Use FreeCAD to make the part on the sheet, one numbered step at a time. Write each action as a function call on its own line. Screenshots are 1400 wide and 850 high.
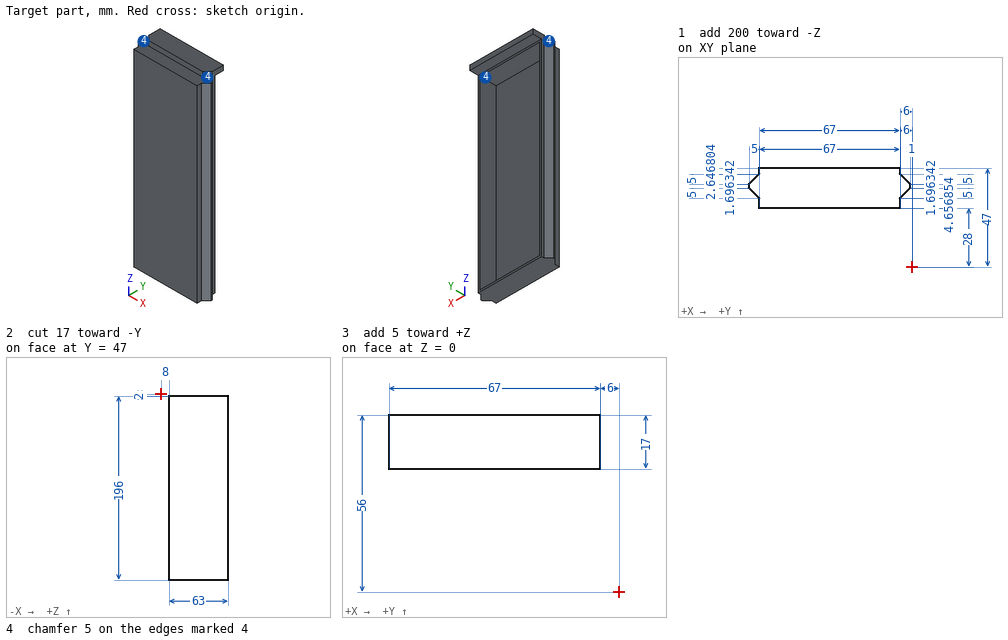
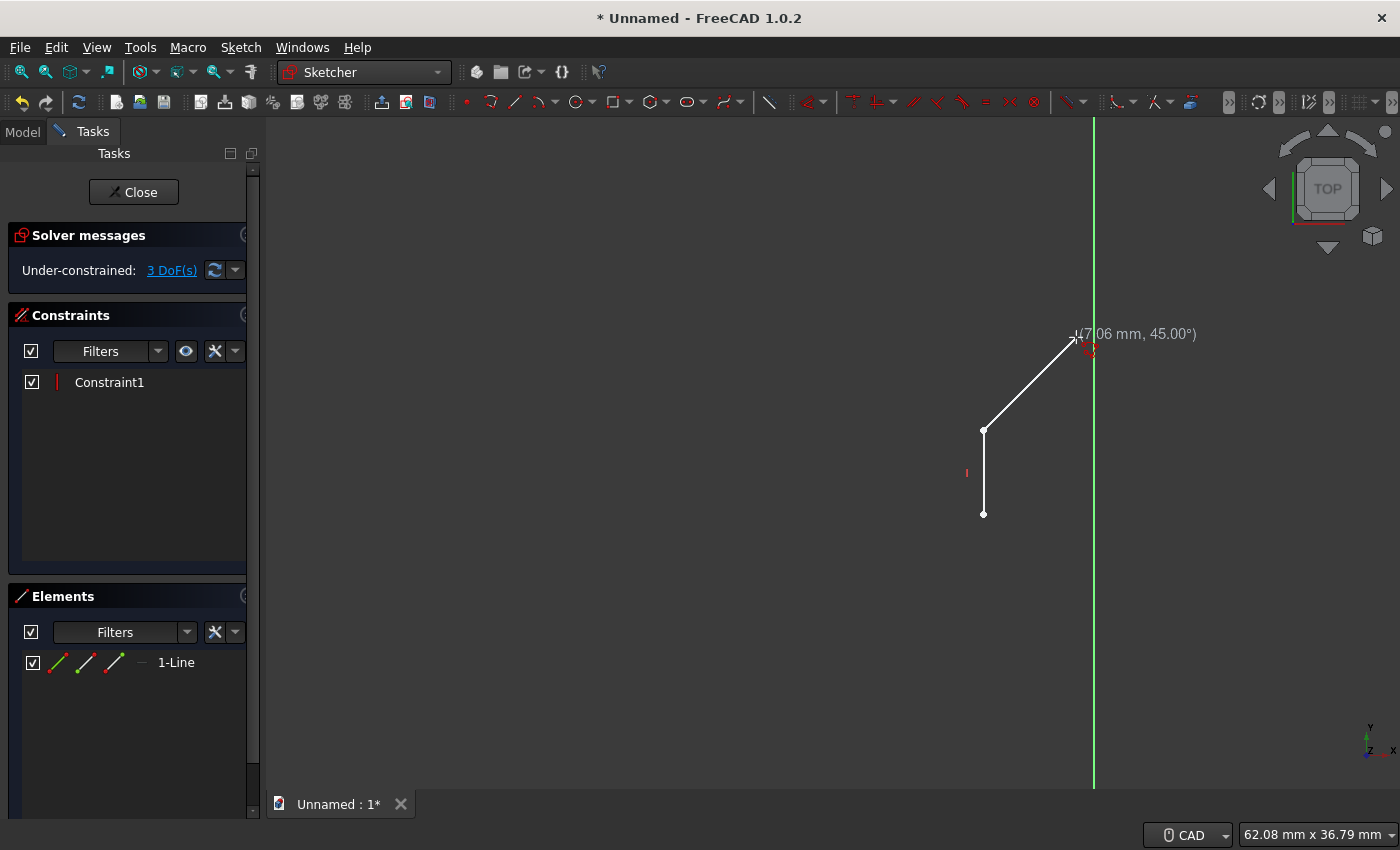
click(1076, 336)
click(1076, 305)
click(984, 213)
click(984, 165)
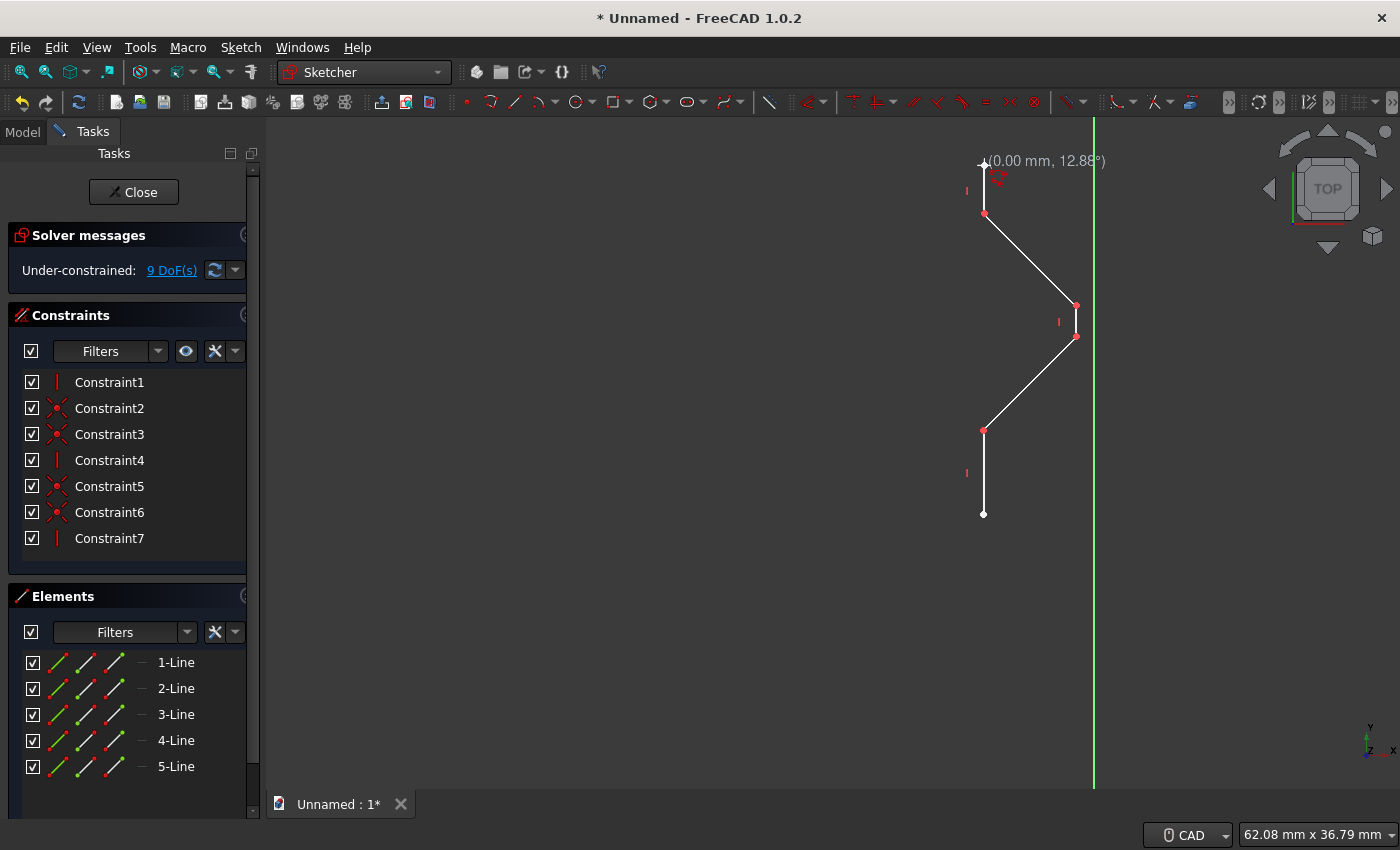
scroll(1077, 338, down, 4)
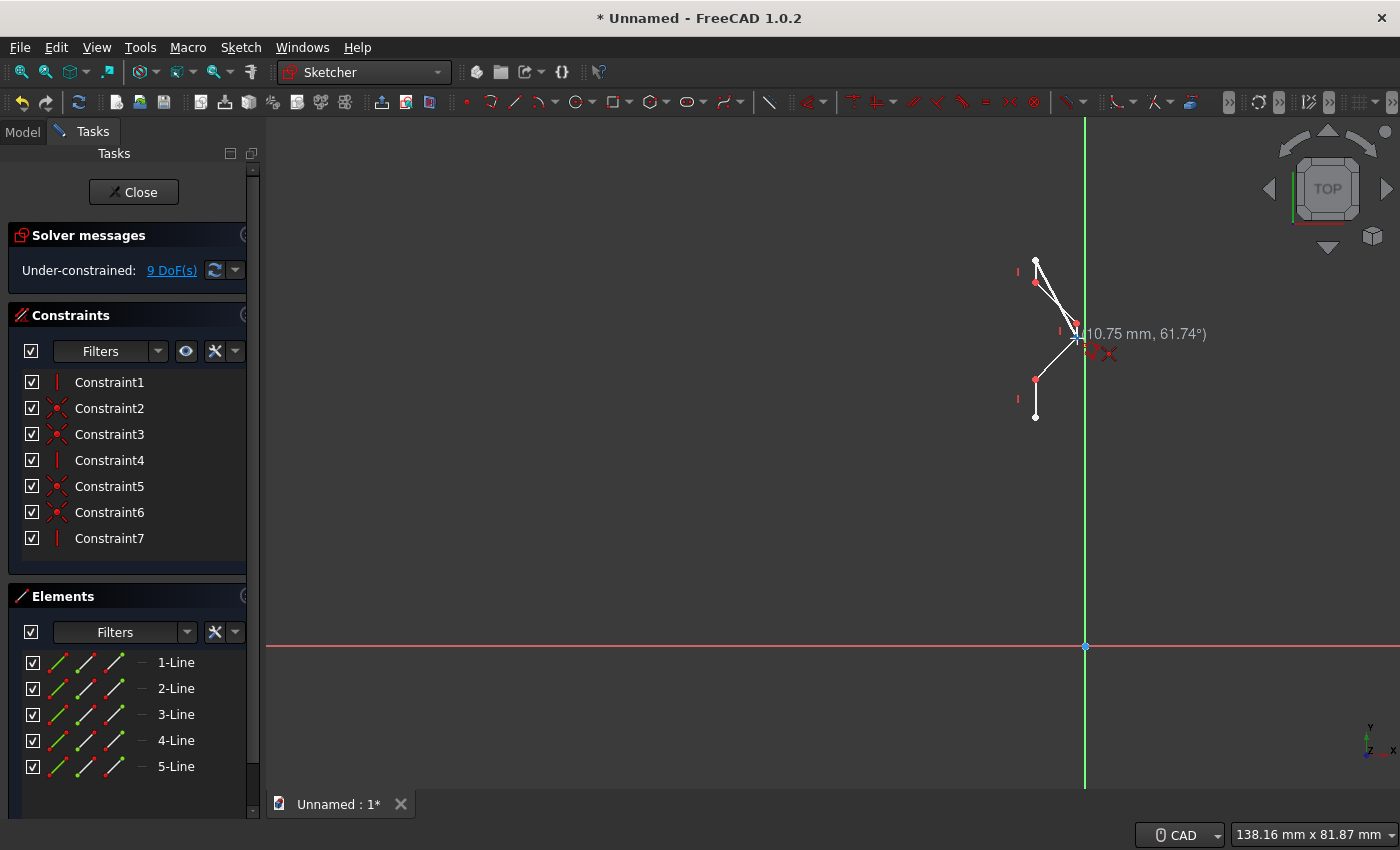
click(486, 260)
click(486, 282)
click(445, 323)
click(445, 337)
click(486, 378)
click(486, 416)
click(1036, 418)
key(Escape)
key(Escape)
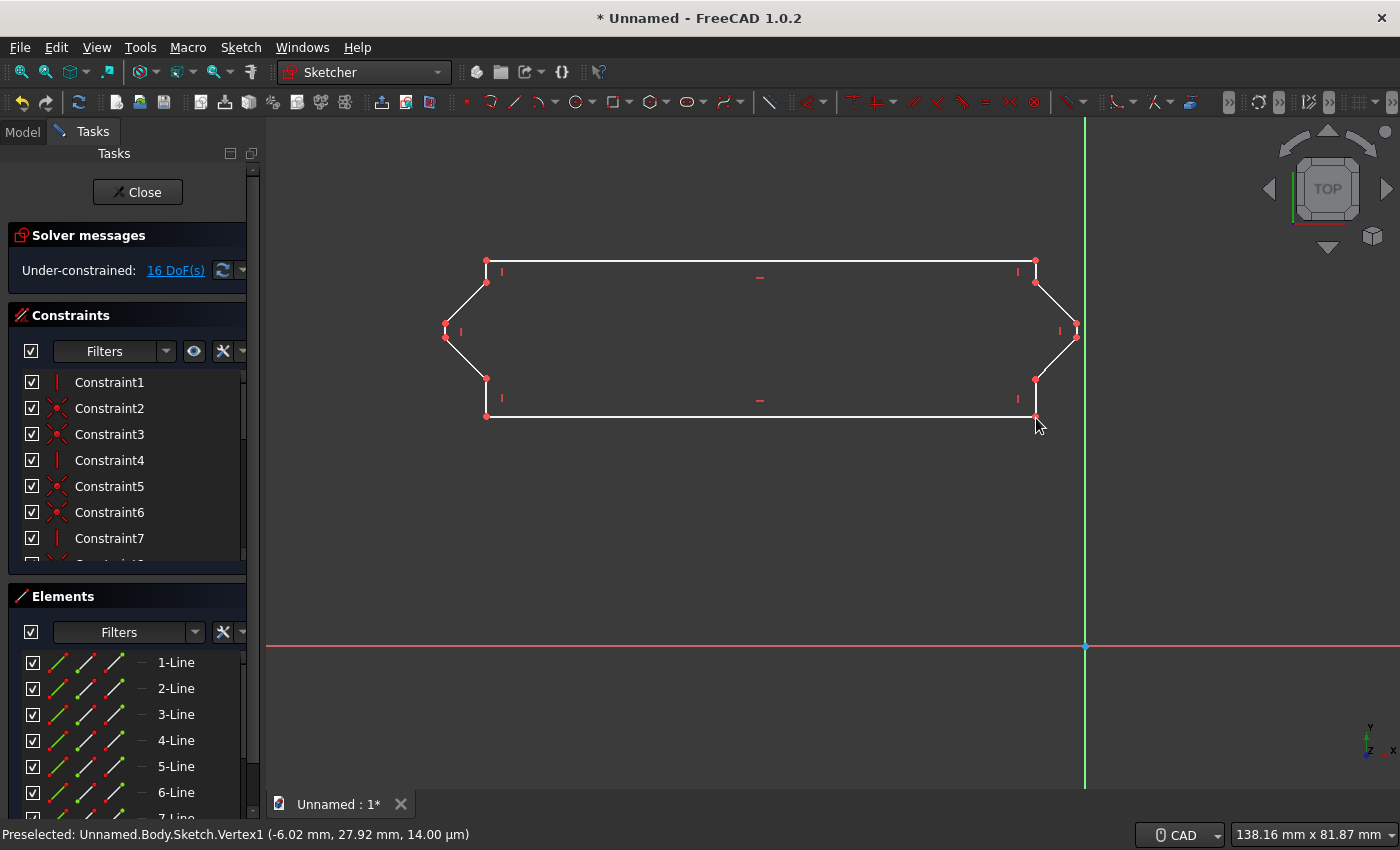
key(d)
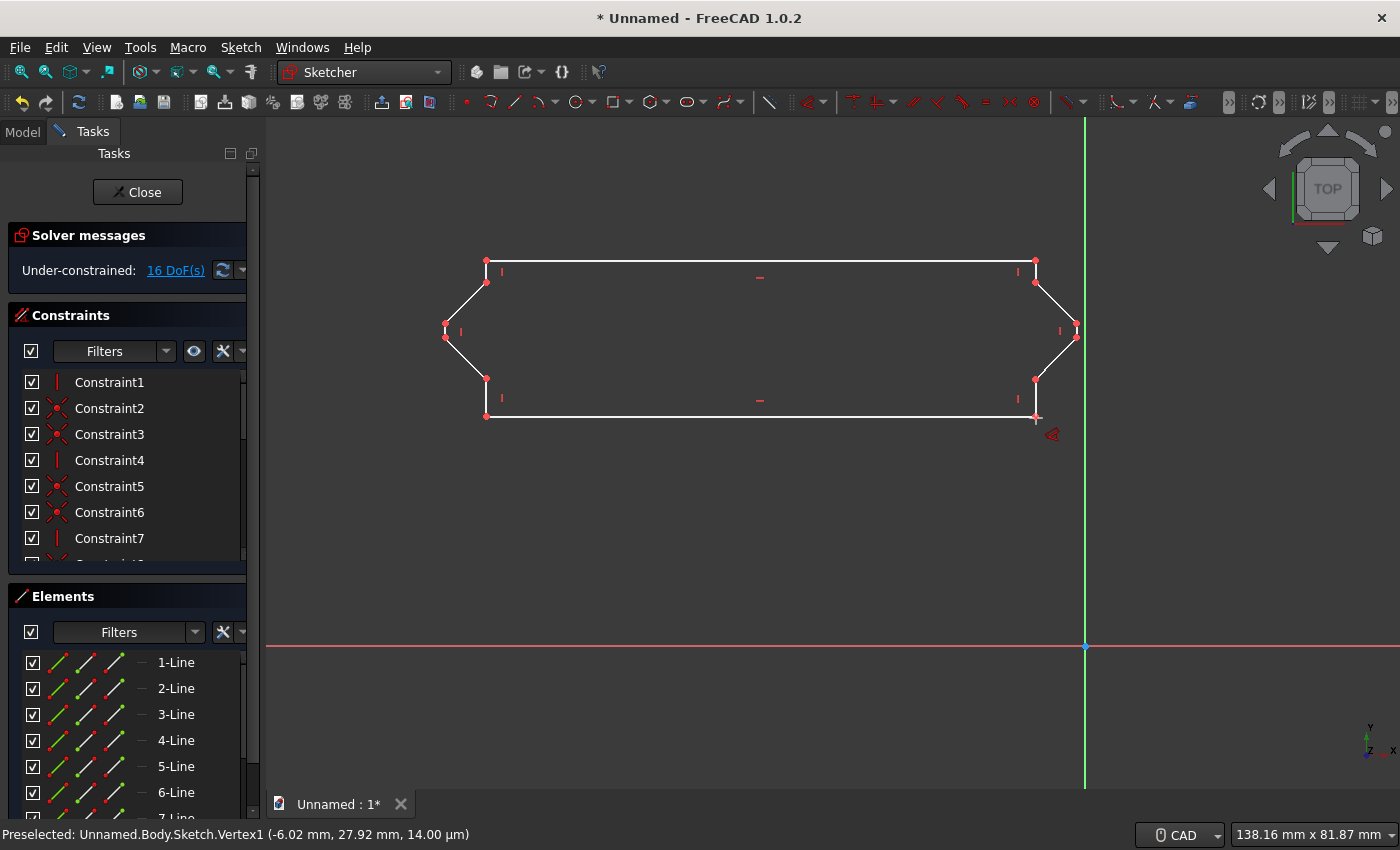
click(871, 261)
click(761, 227)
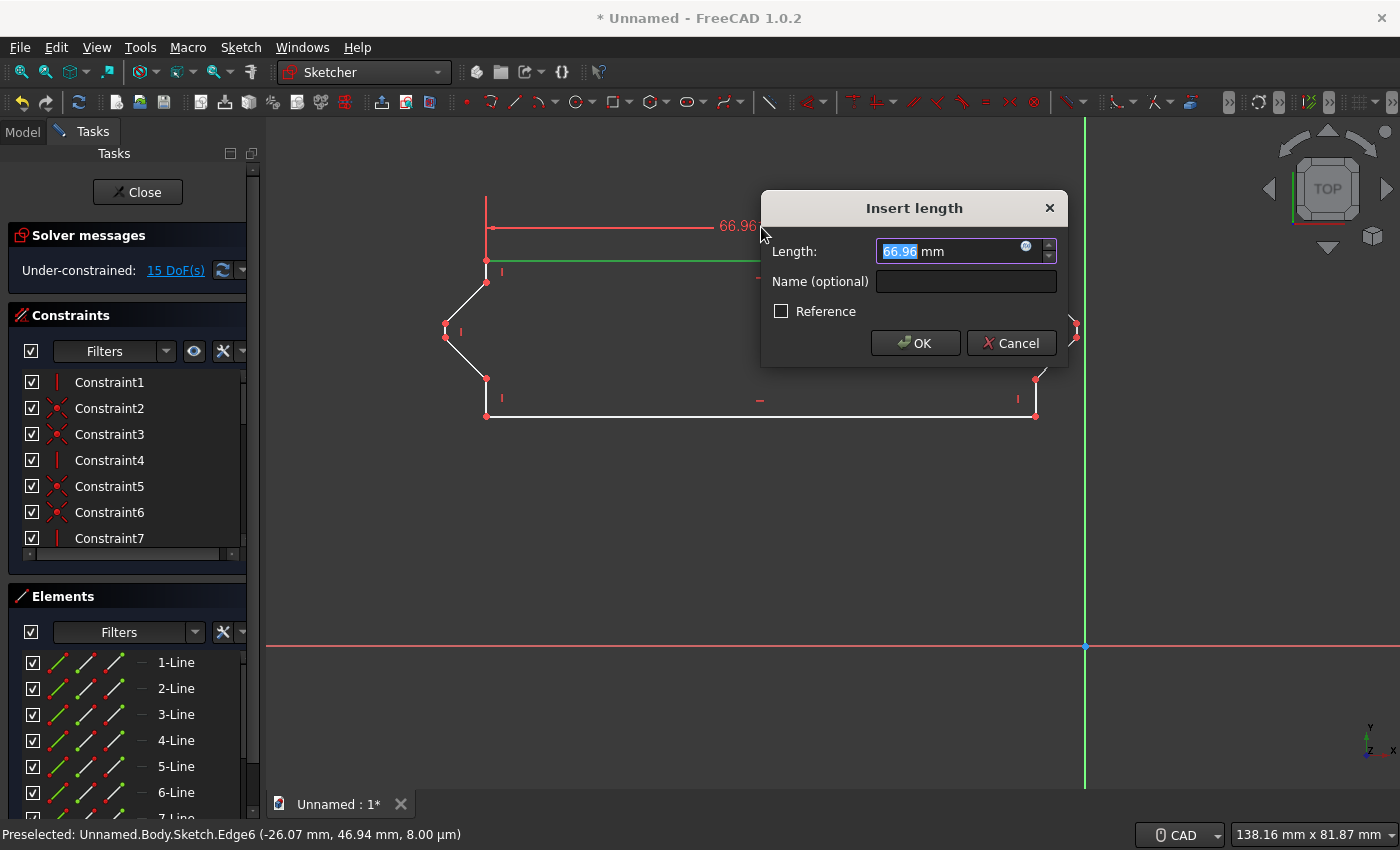
text(67)
key(Return)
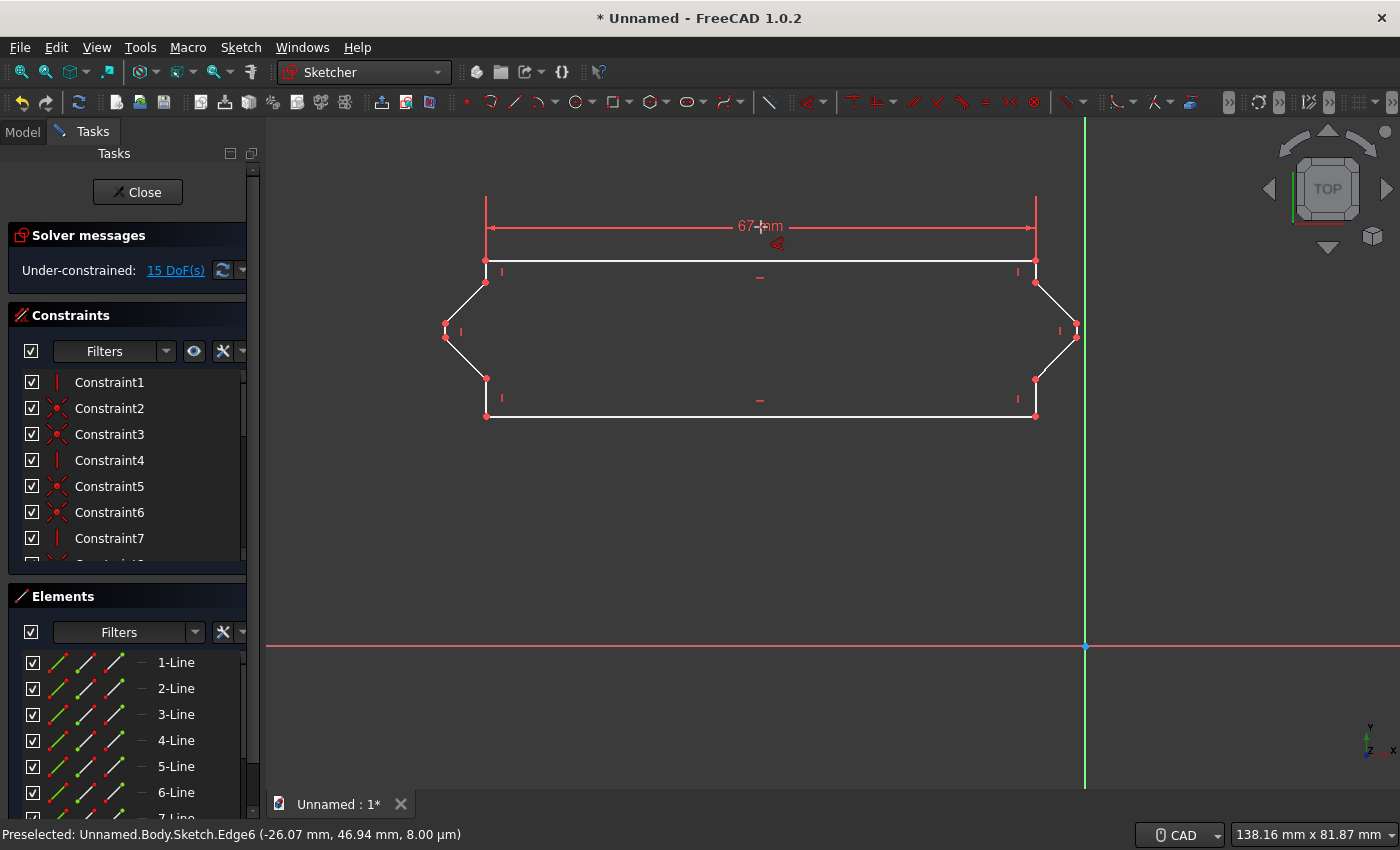
click(651, 417)
click(761, 383)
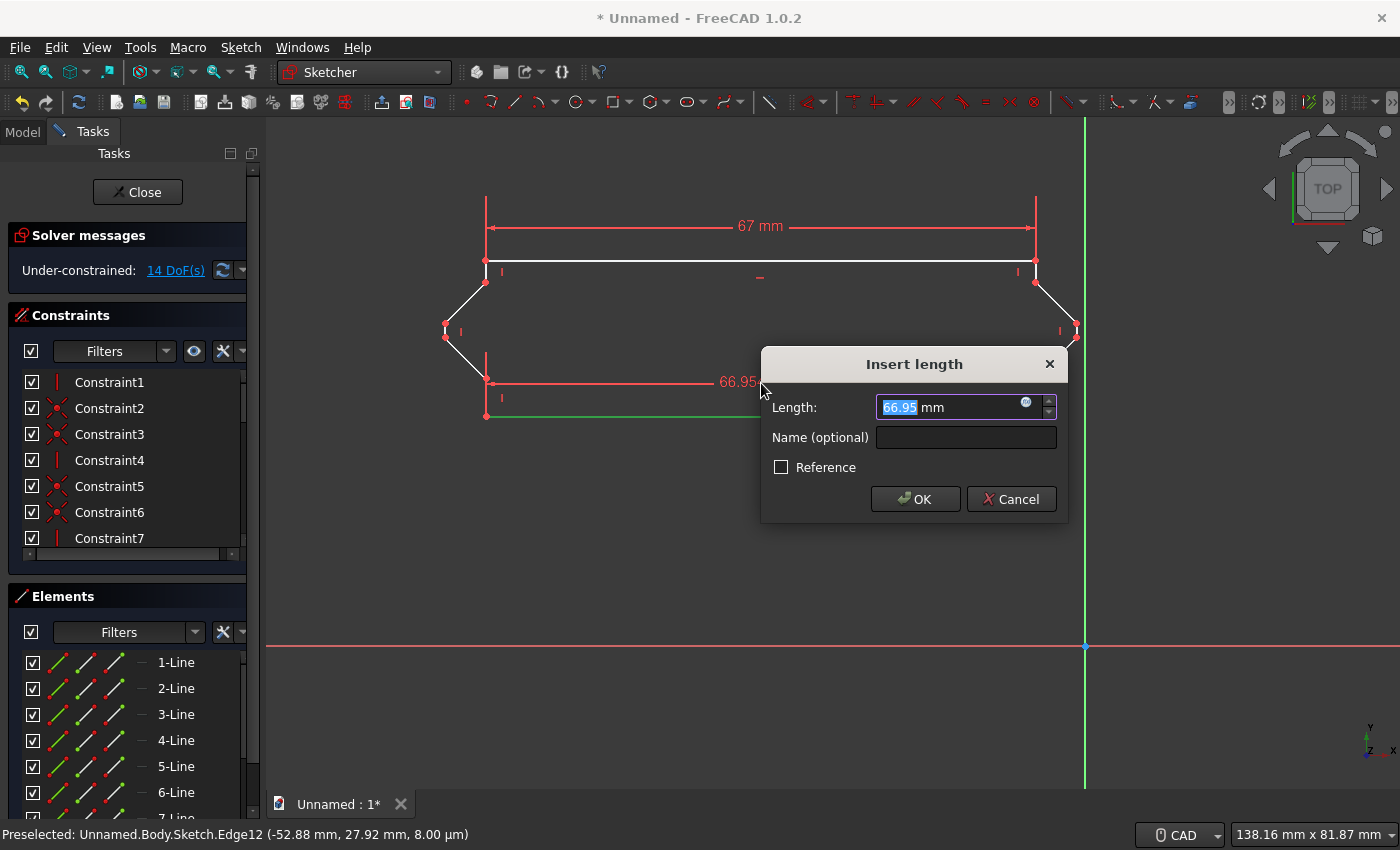
text(67)
key(Return)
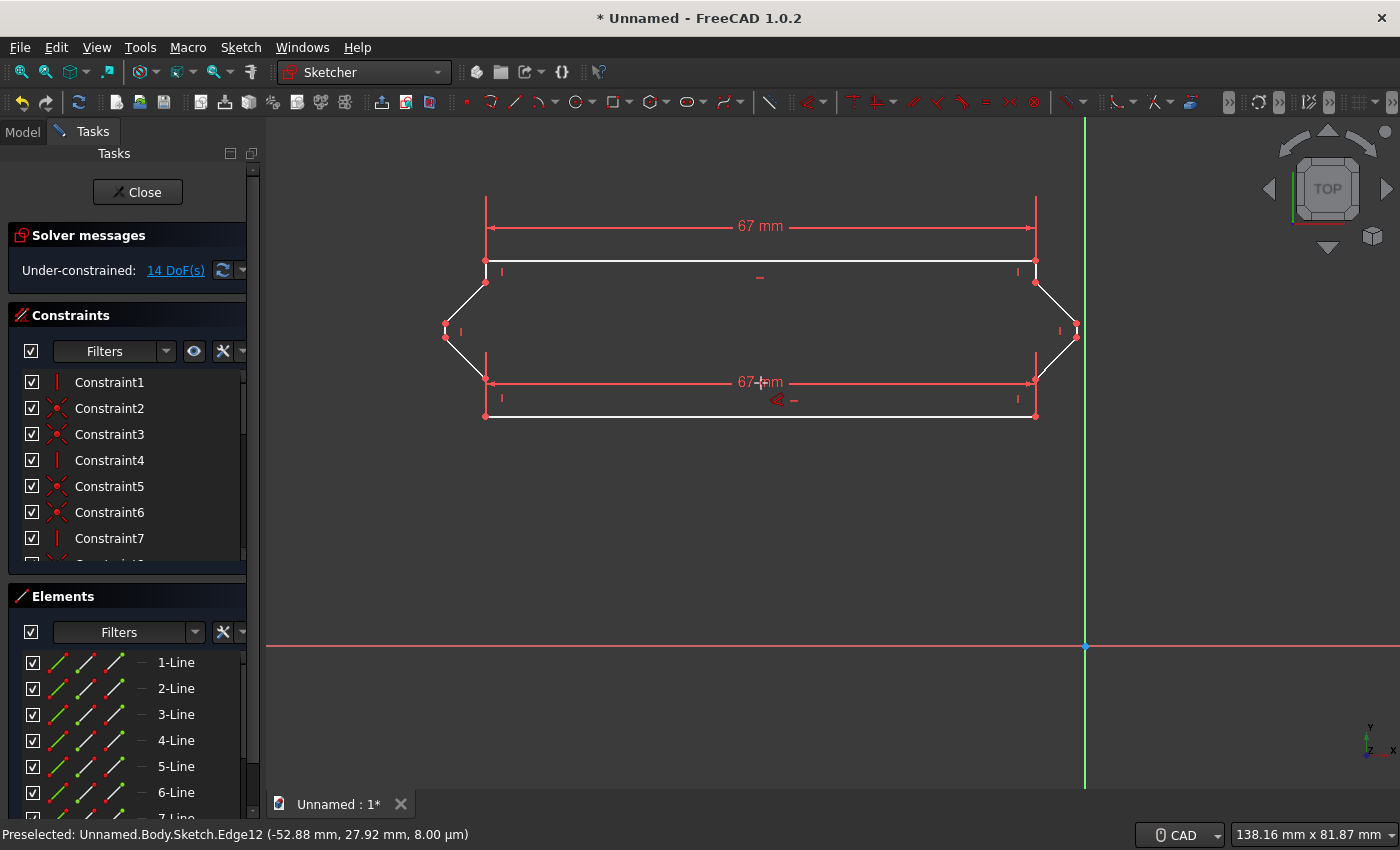
click(1036, 417)
click(1060, 680)